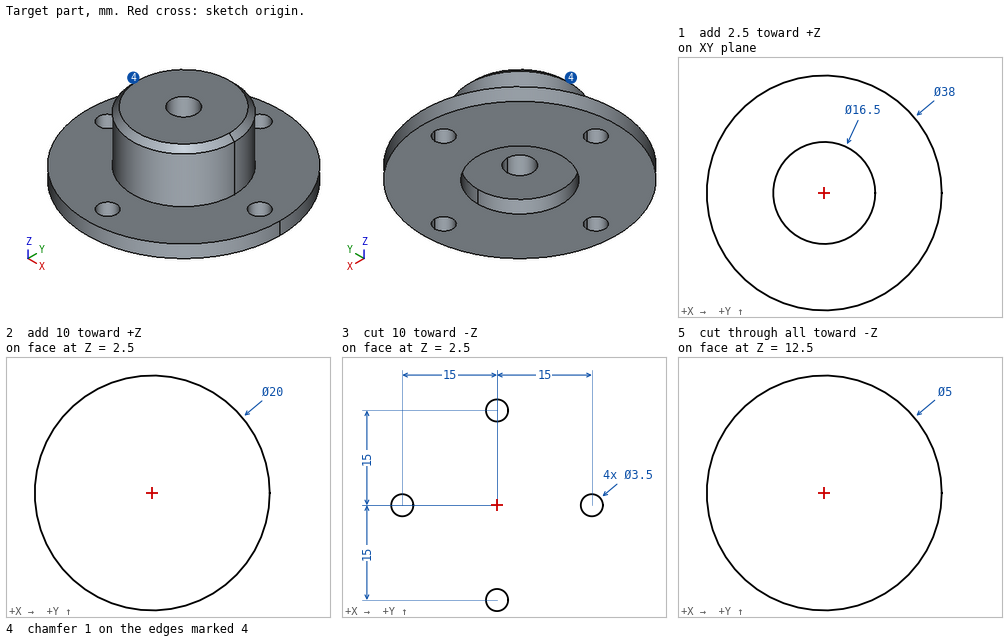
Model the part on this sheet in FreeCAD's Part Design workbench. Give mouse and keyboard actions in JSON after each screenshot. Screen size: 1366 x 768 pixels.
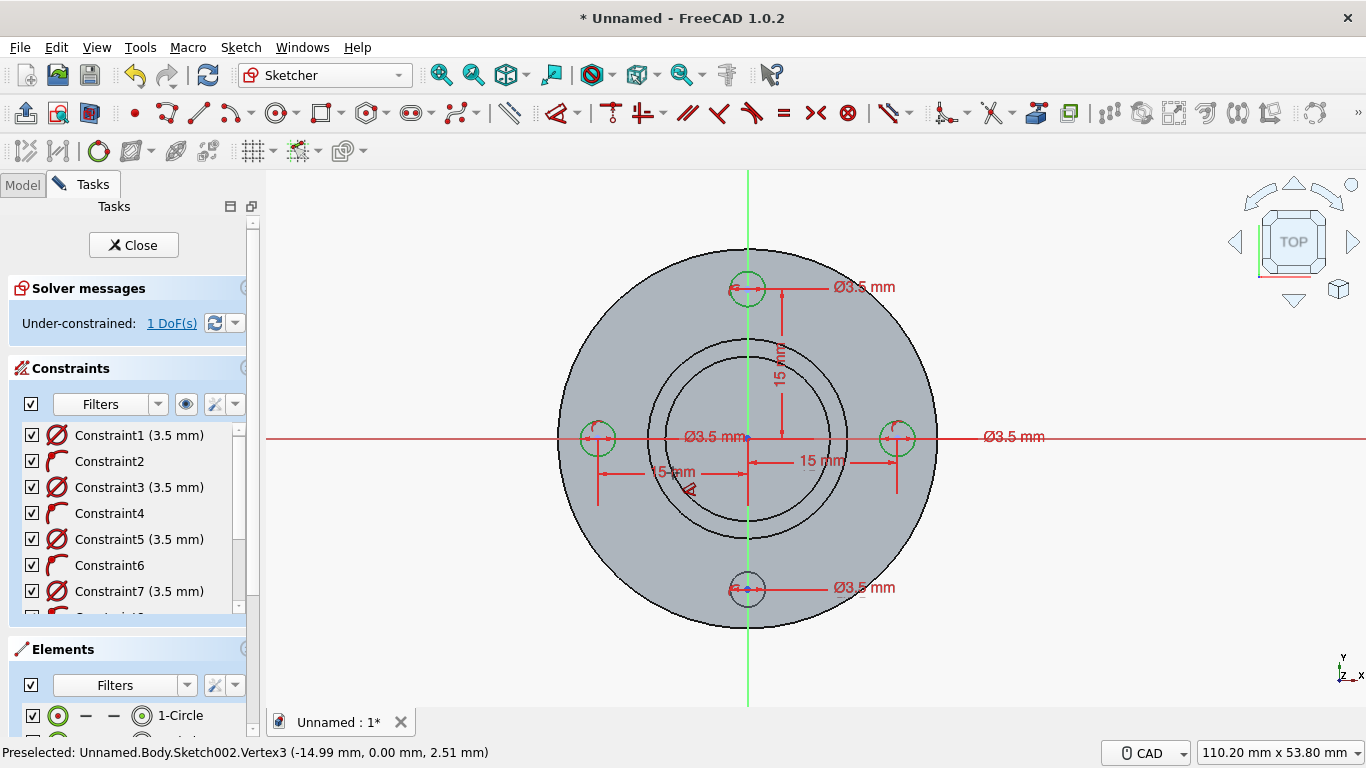
{"action": "left_click", "coordinate": [748, 590]}
{"action": "left_click", "coordinate": [782, 514]}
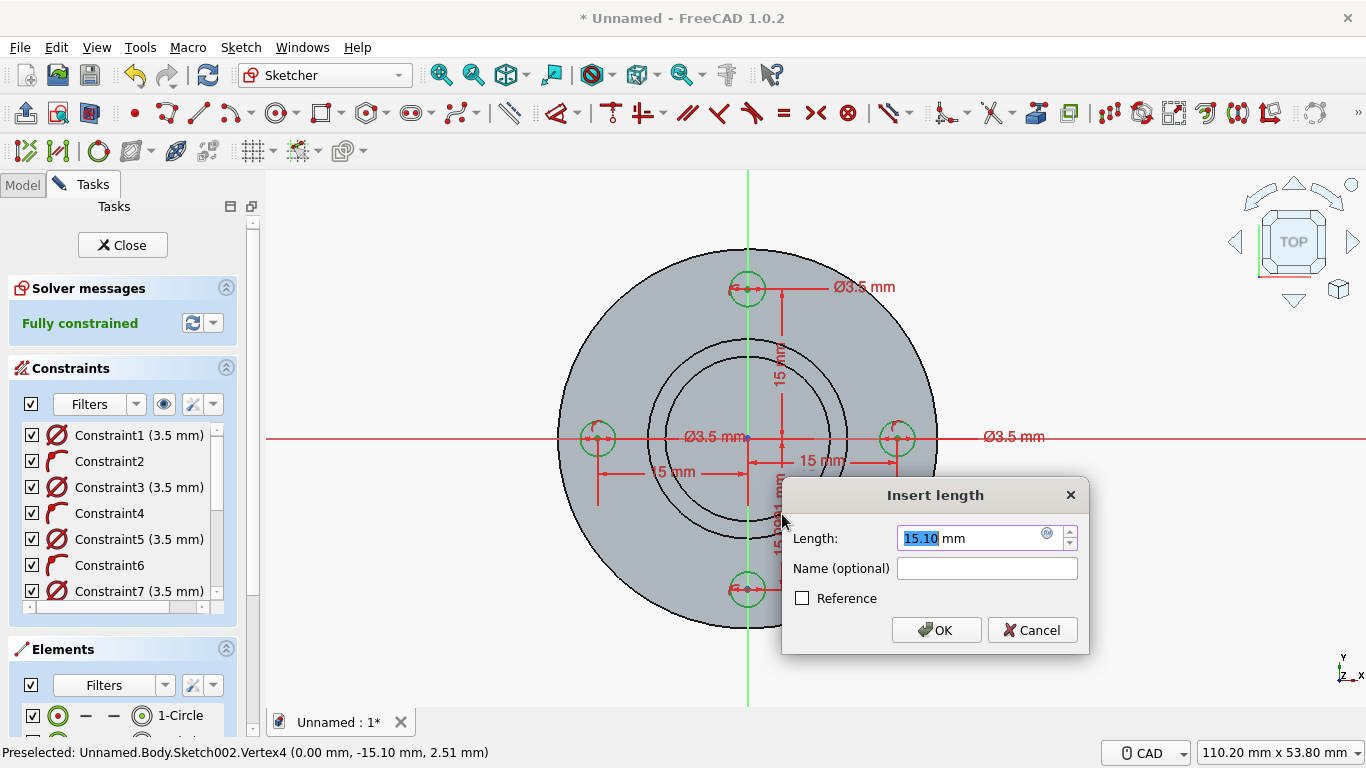
{"action": "type", "text": "15"}
{"action": "key", "text": "Return"}
{"action": "key", "text": "Escape"}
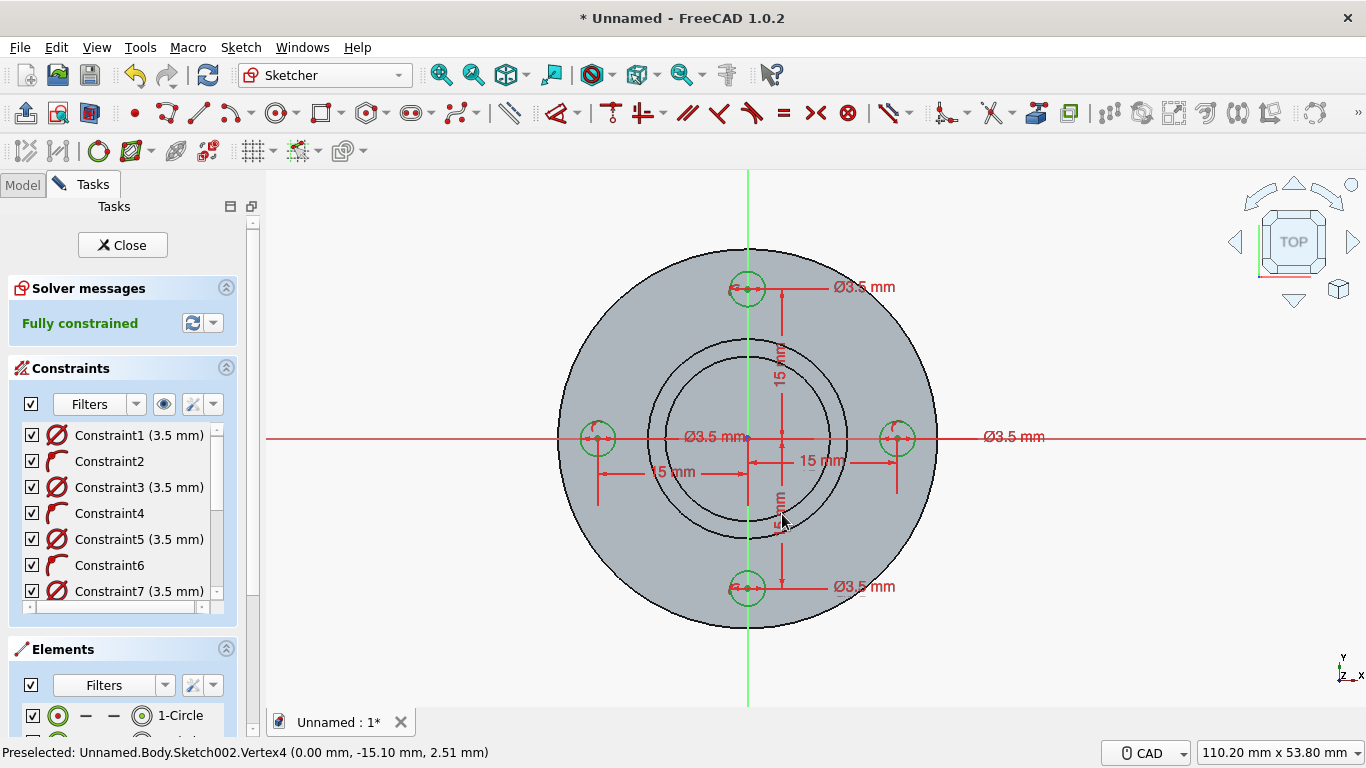
{"action": "left_click", "coordinate": [123, 245]}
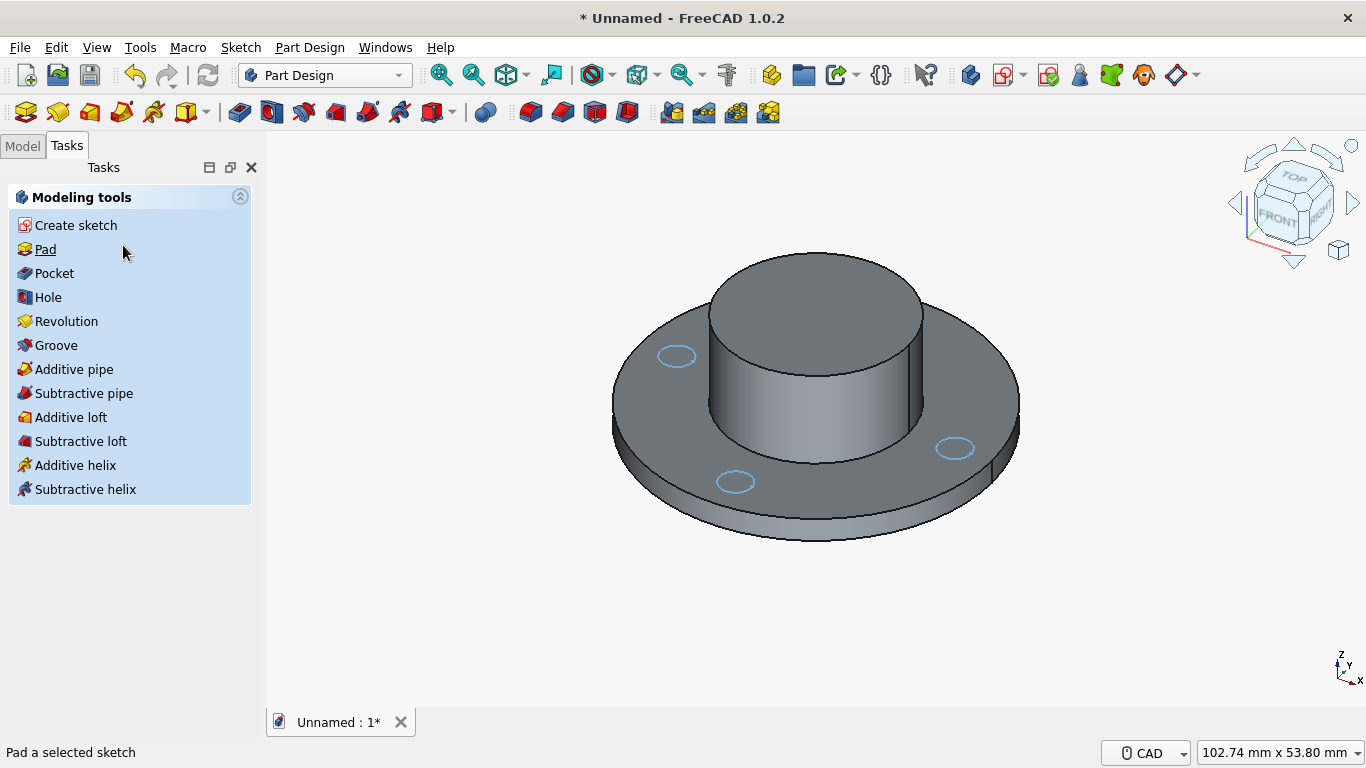
{"action": "left_click", "coordinate": [240, 112]}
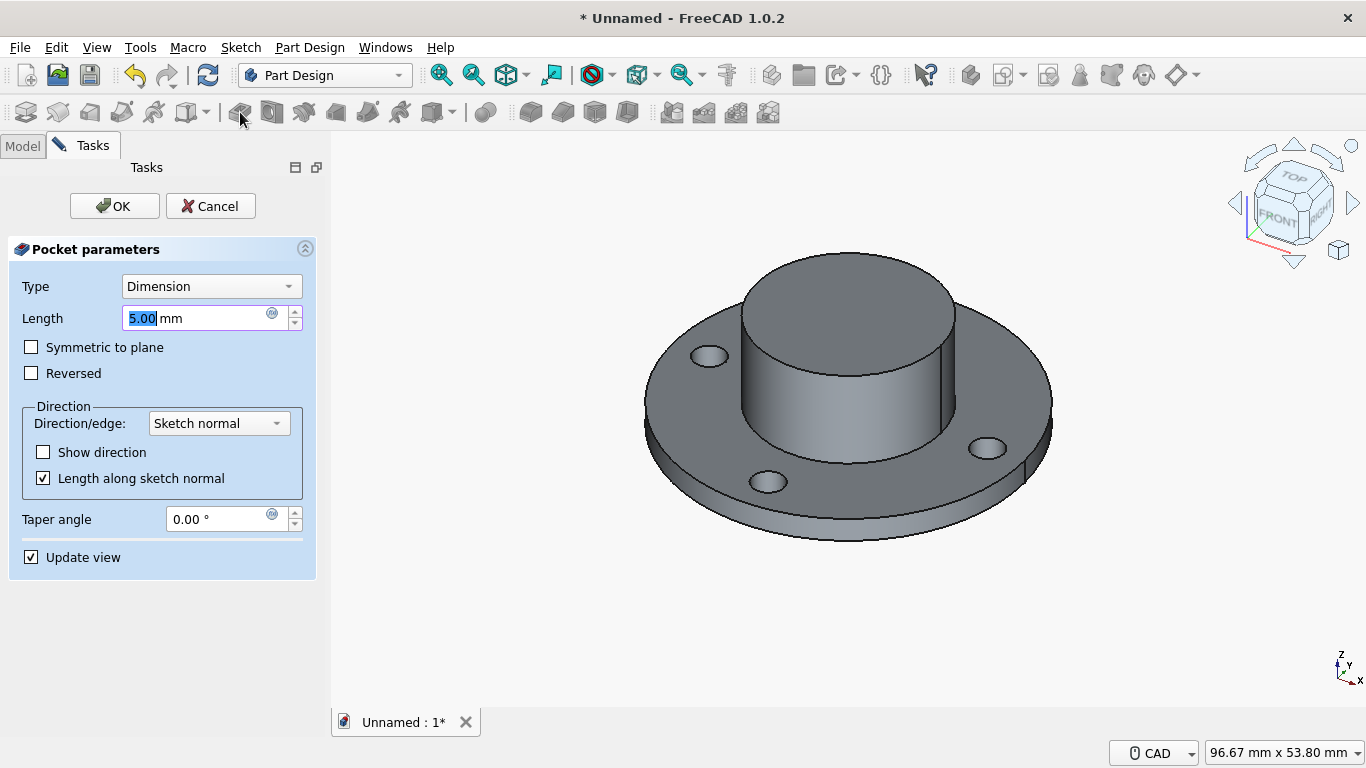
{"action": "type", "text": "10"}
{"action": "key", "text": "Tab"}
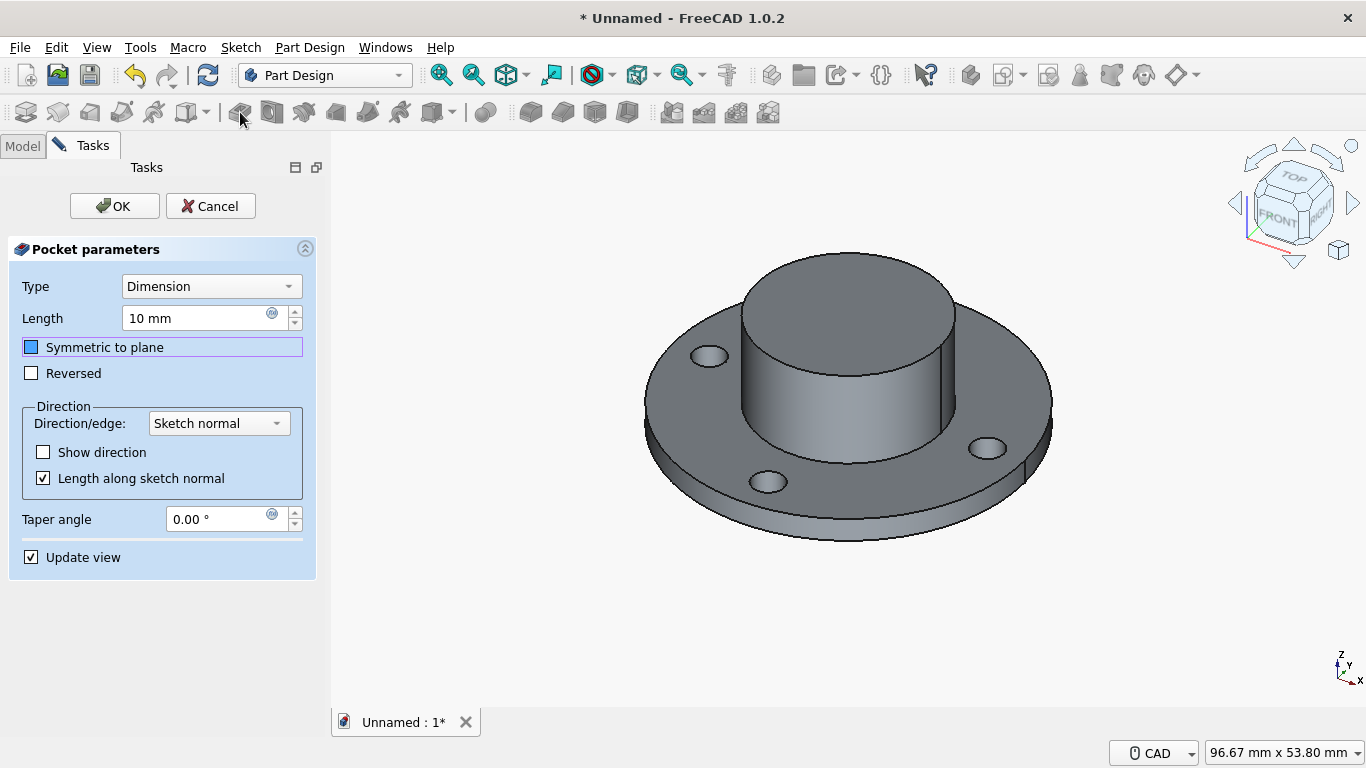
{"action": "left_click", "coordinate": [115, 206]}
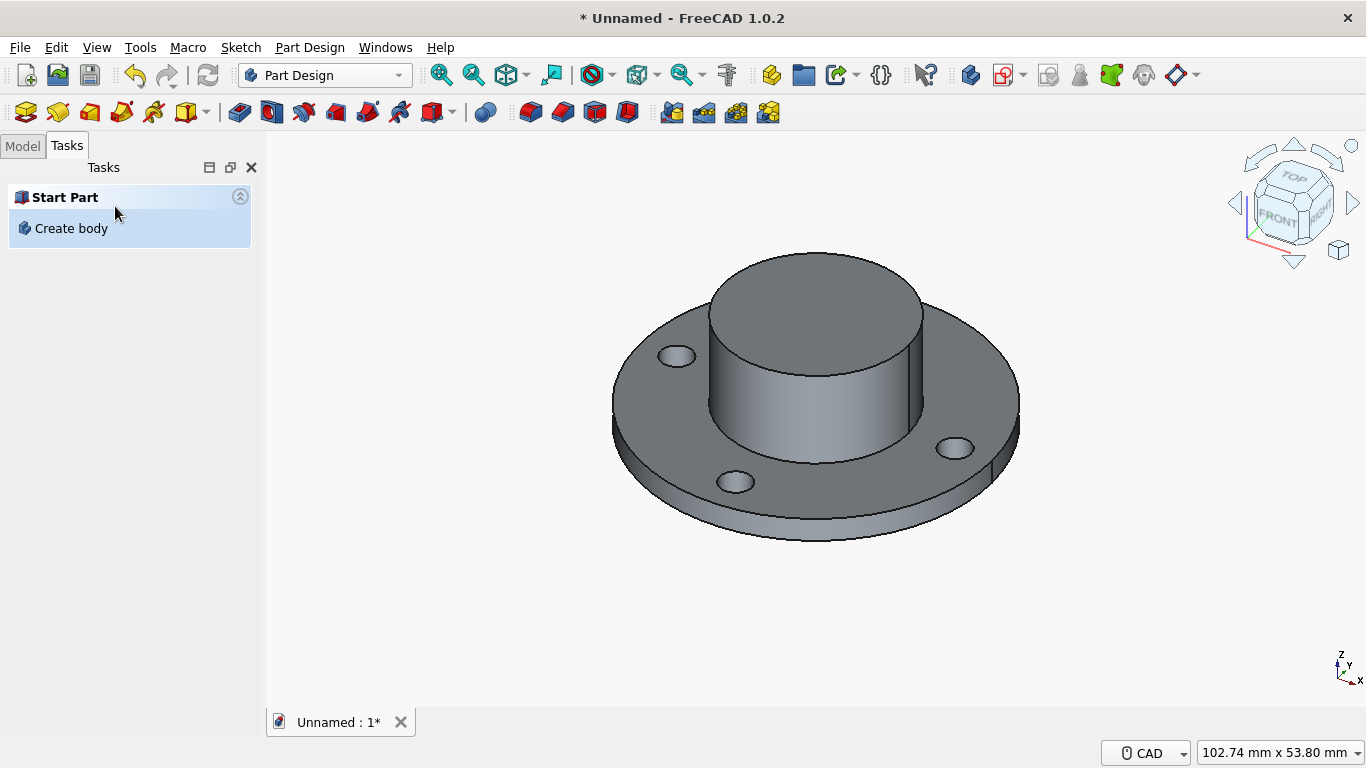
{"action": "left_click", "coordinate": [710, 320]}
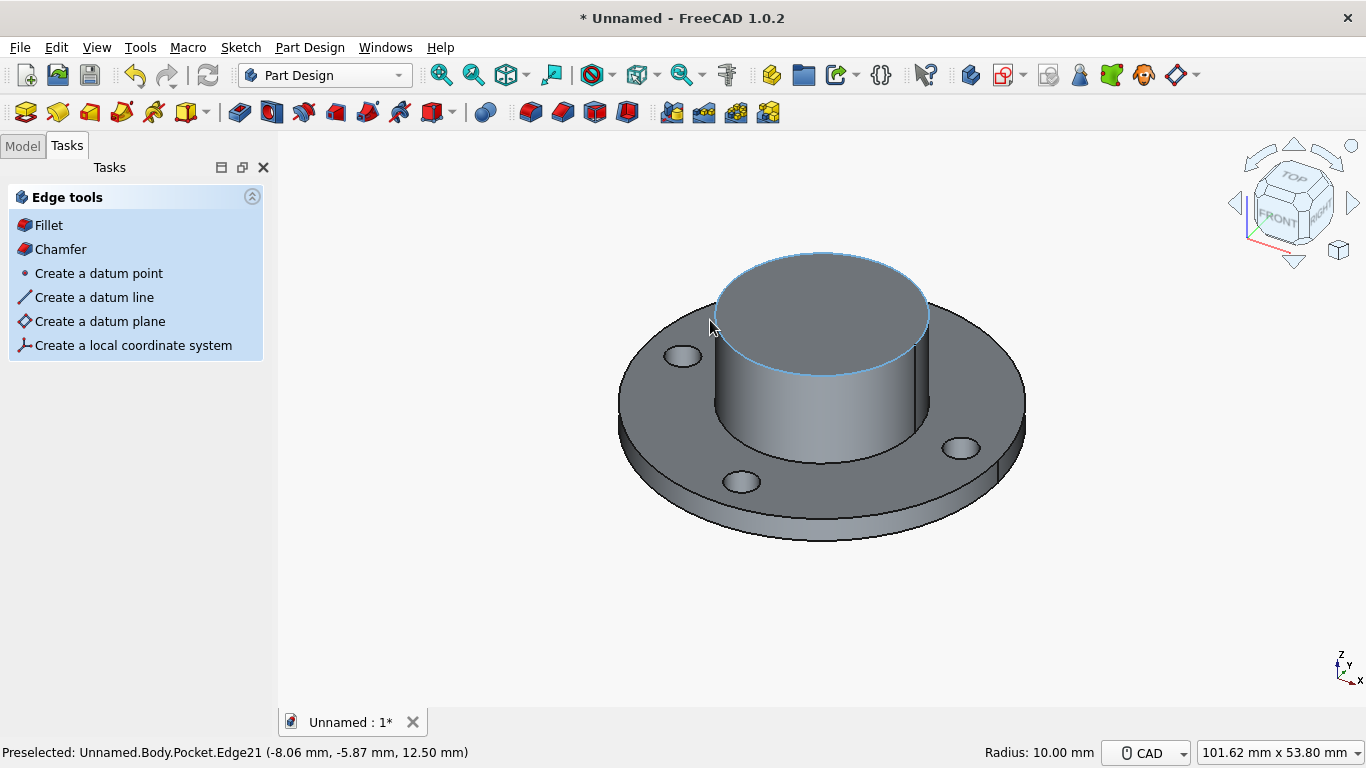
{"action": "left_click", "coordinate": [564, 112]}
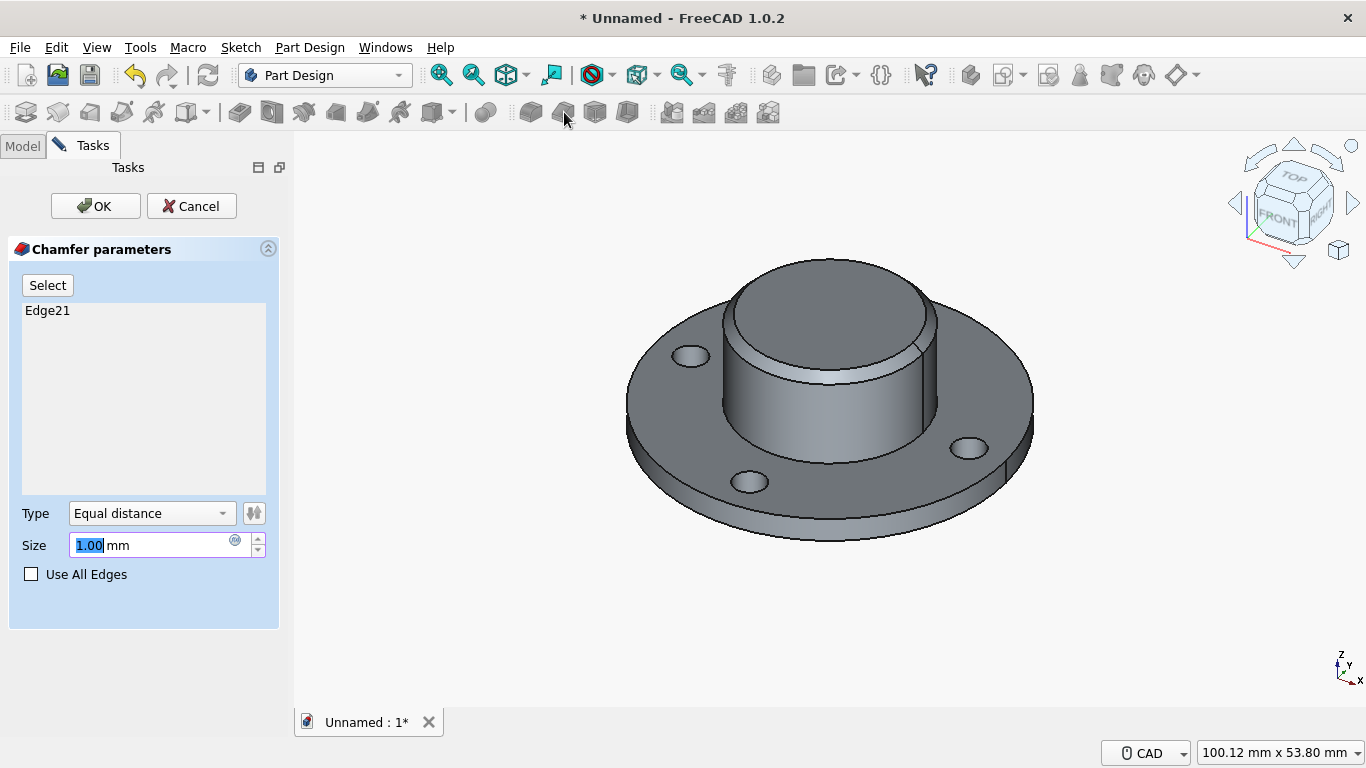
{"action": "type", "text": "1"}
{"action": "key", "text": "Tab"}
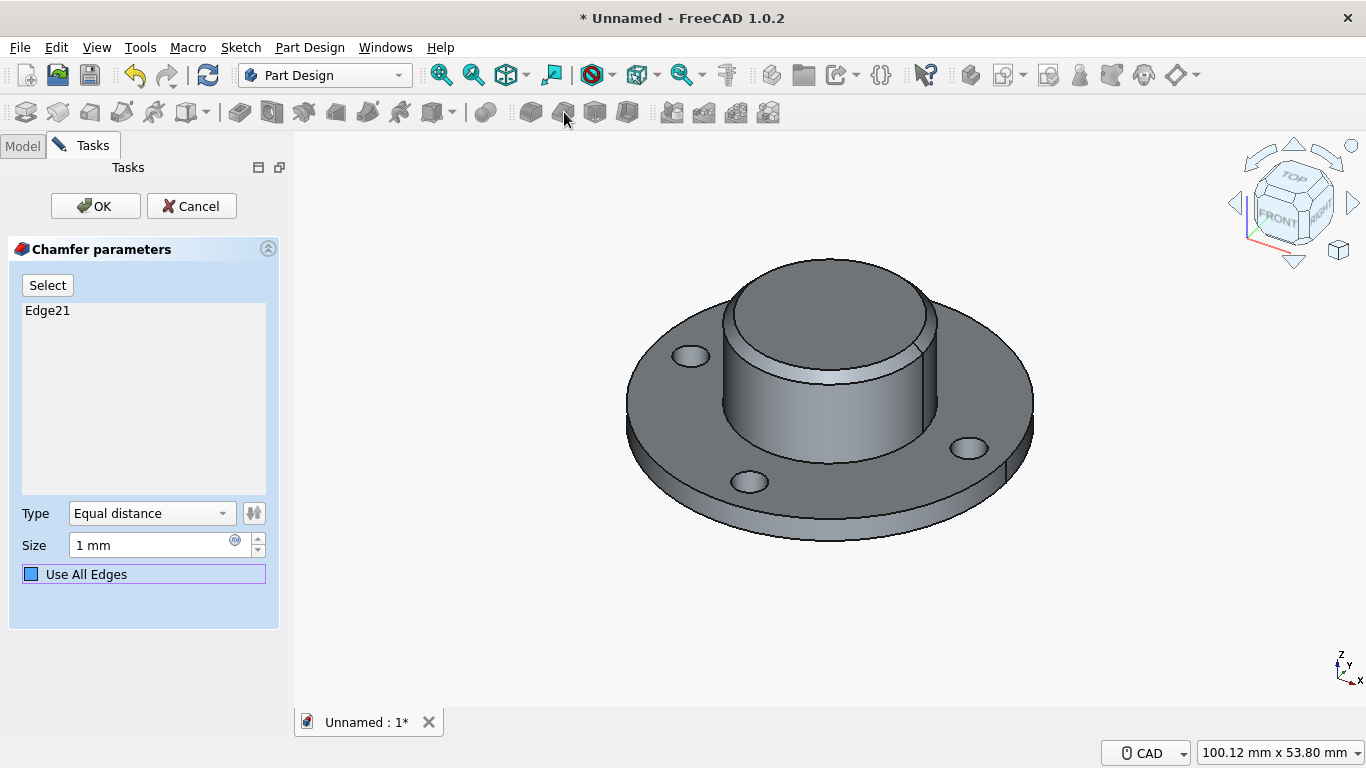
{"action": "left_click", "coordinate": [96, 206]}